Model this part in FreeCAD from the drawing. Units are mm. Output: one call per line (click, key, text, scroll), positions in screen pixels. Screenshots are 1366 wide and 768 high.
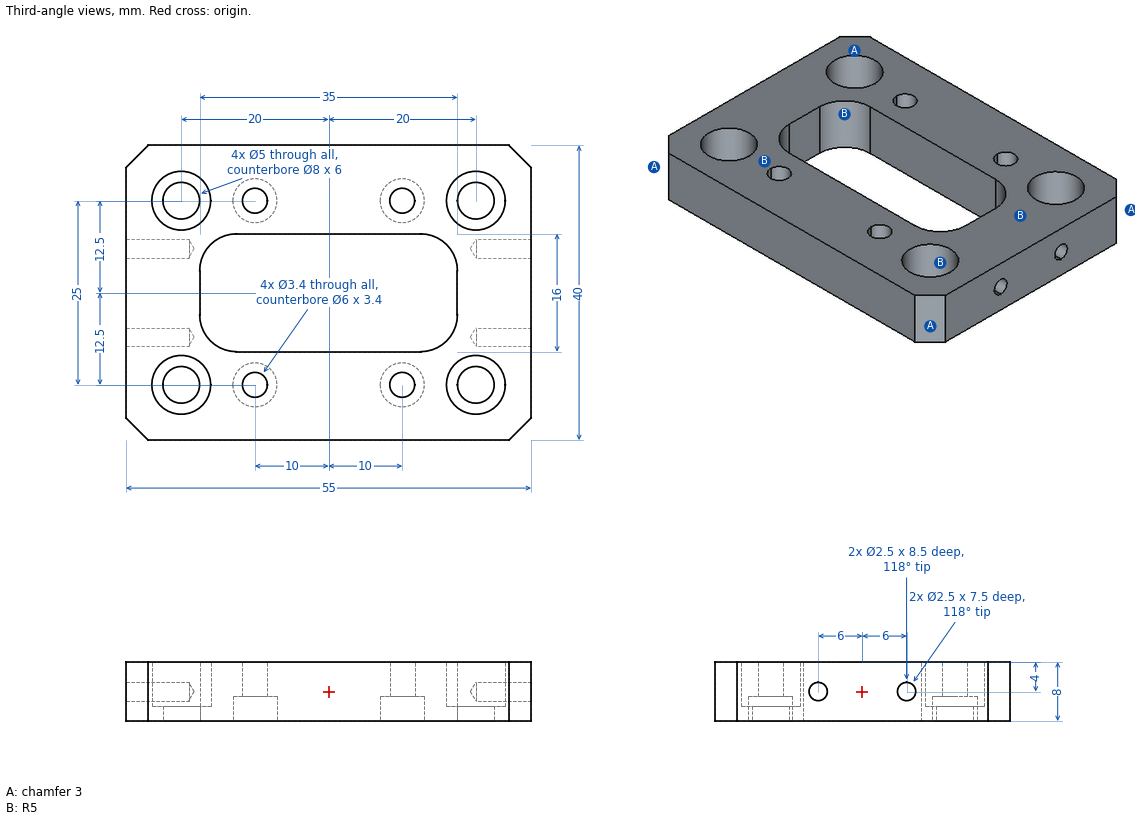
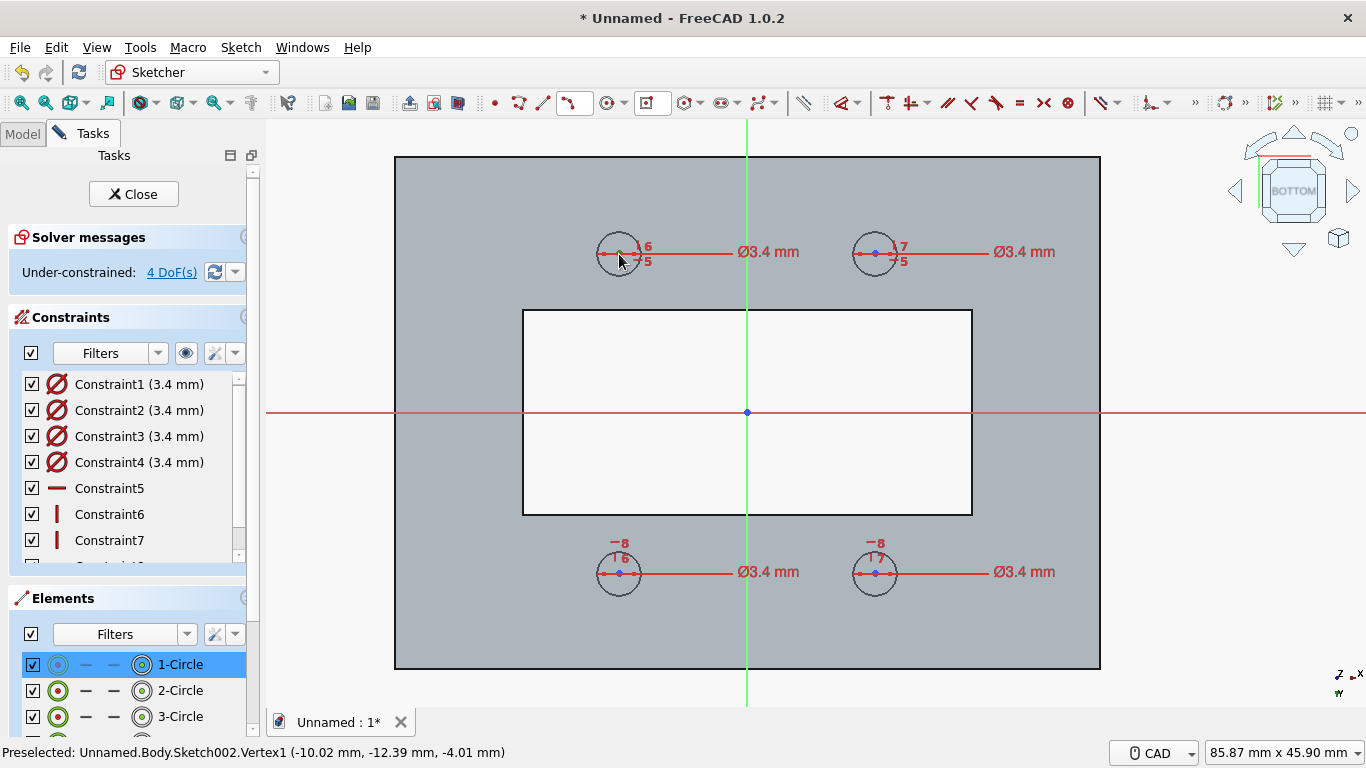
click(860, 104)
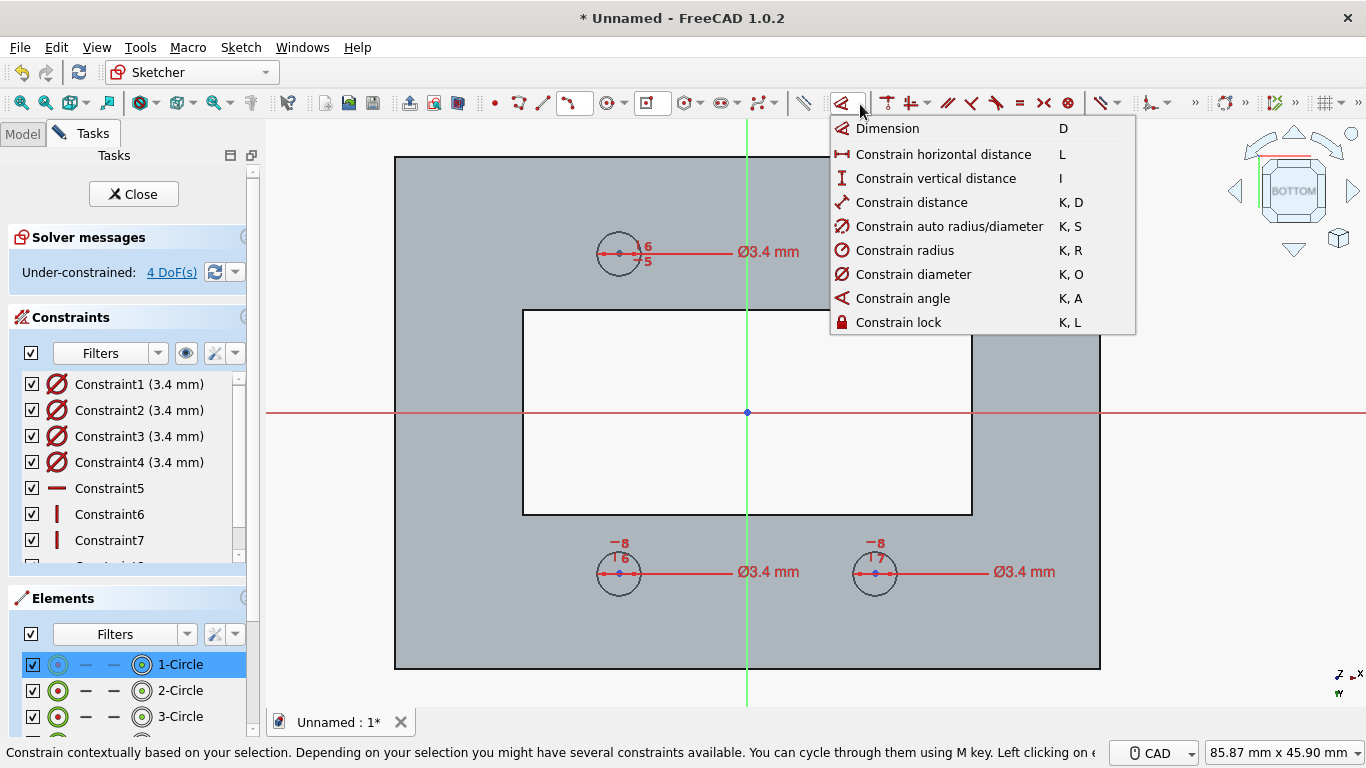
click(983, 154)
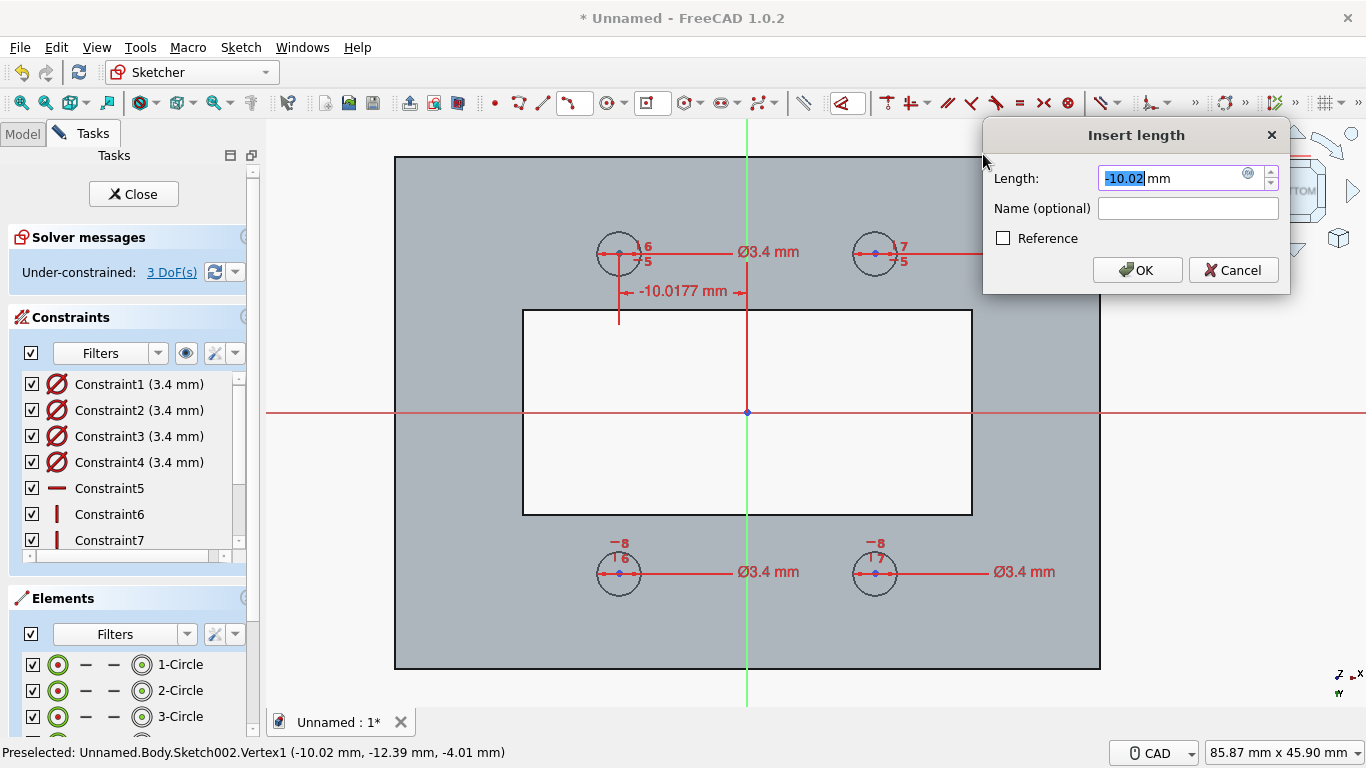
text(-10)
key(Return)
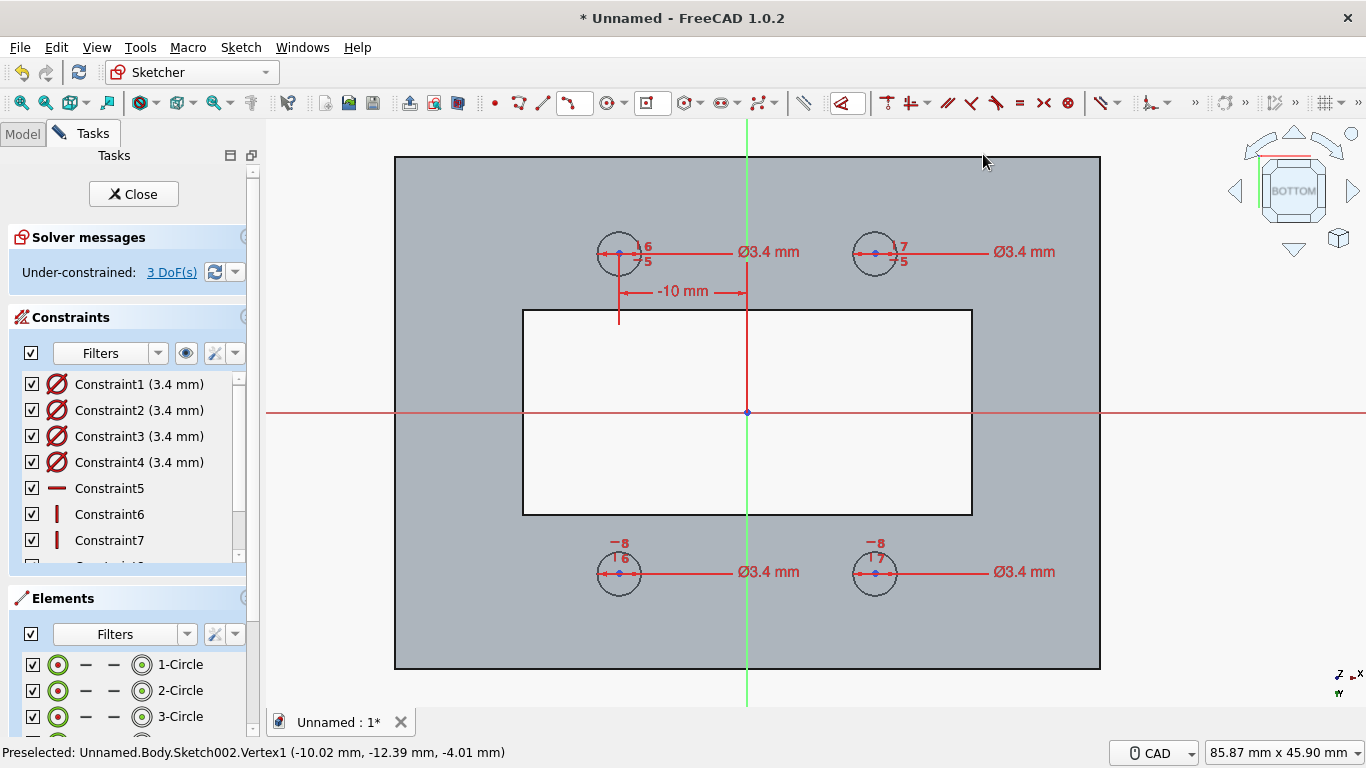
click(875, 254)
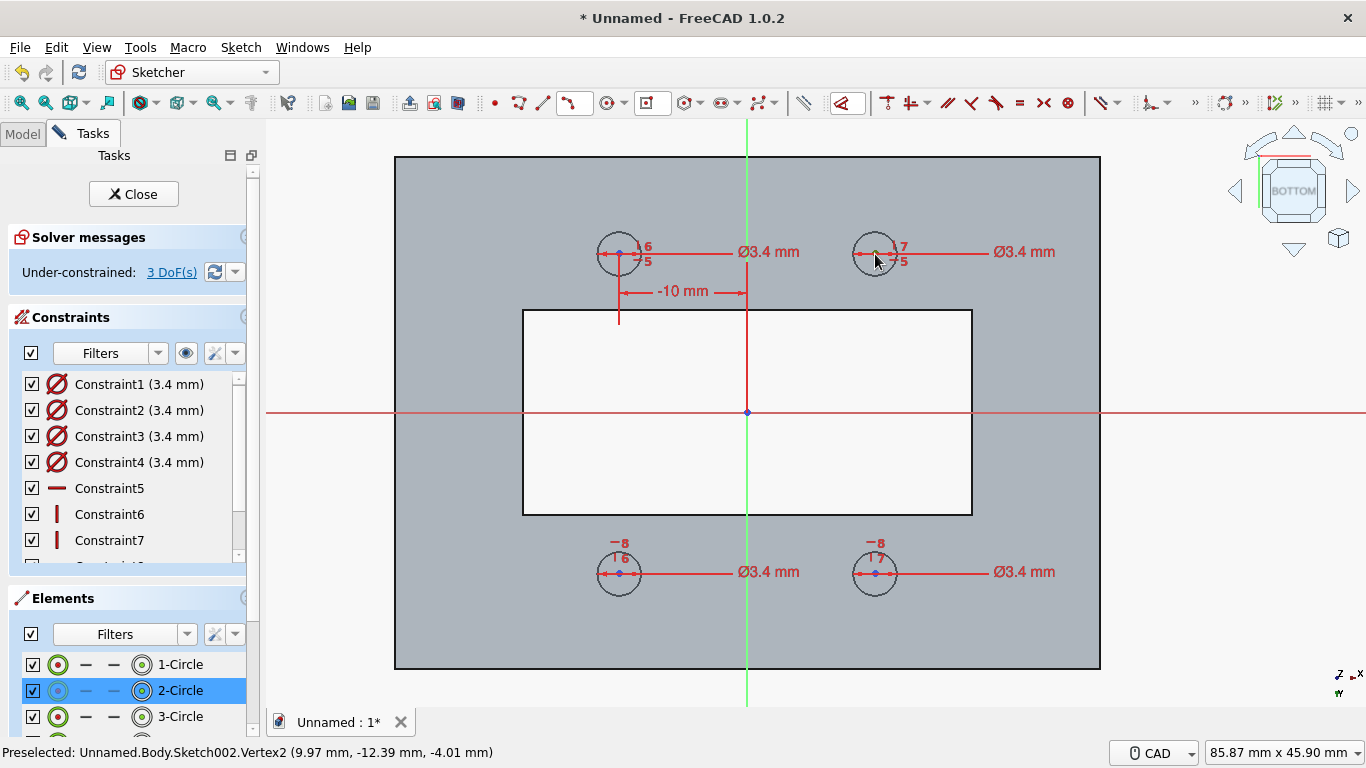
click(860, 104)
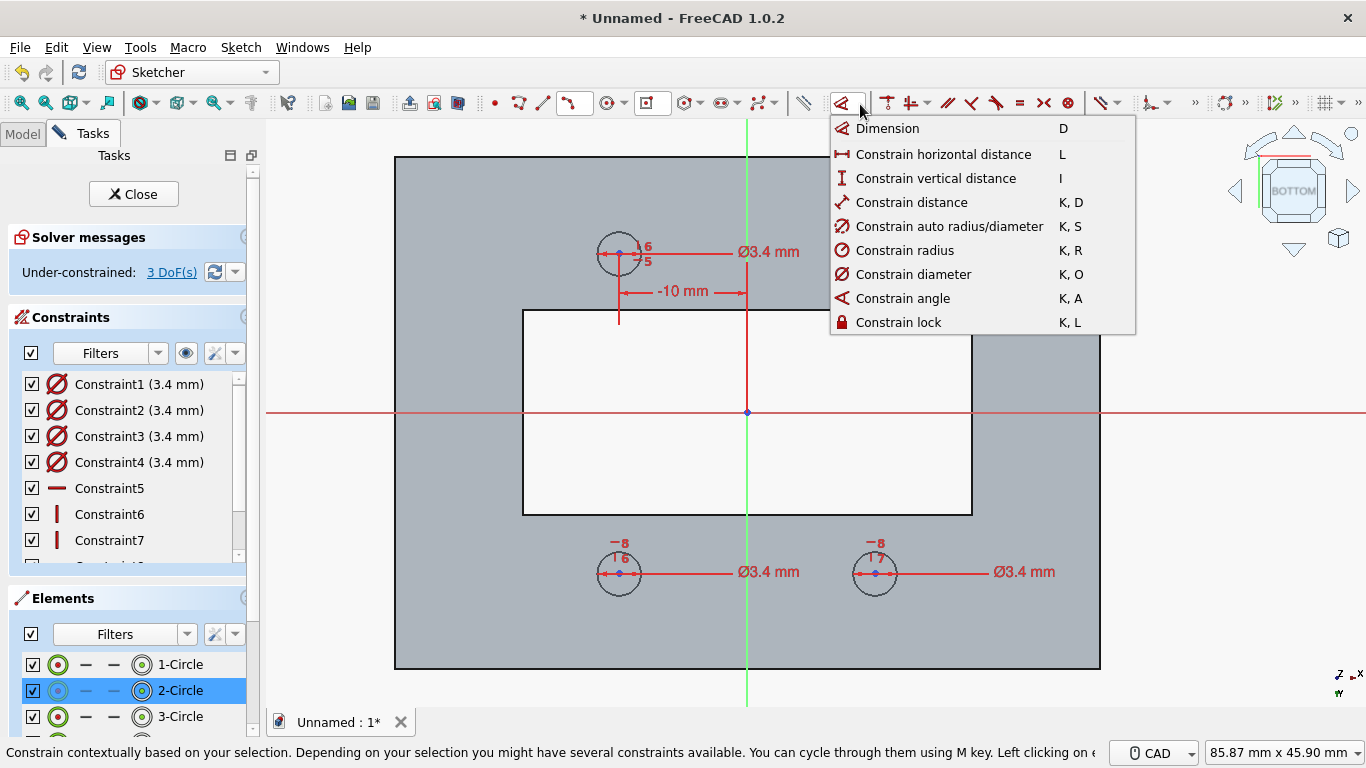
click(983, 154)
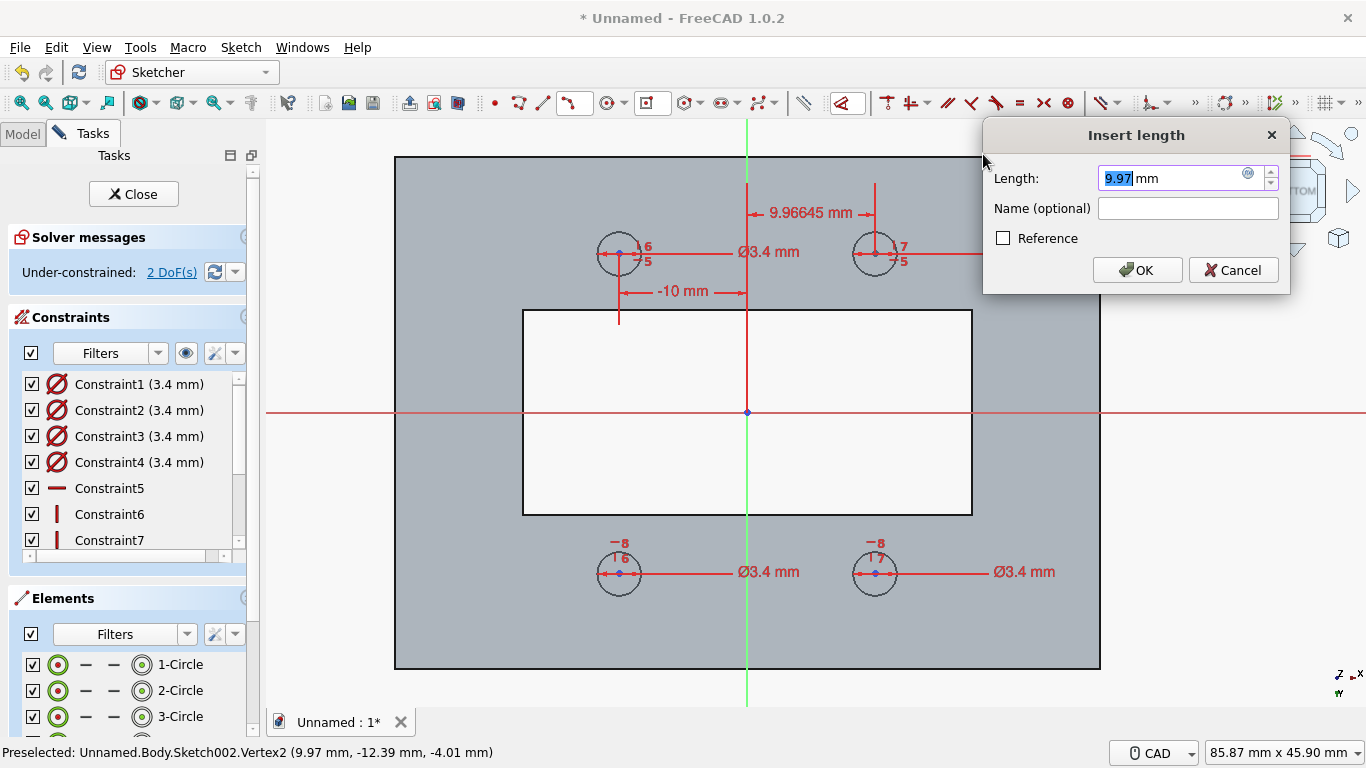
text(10)
key(Return)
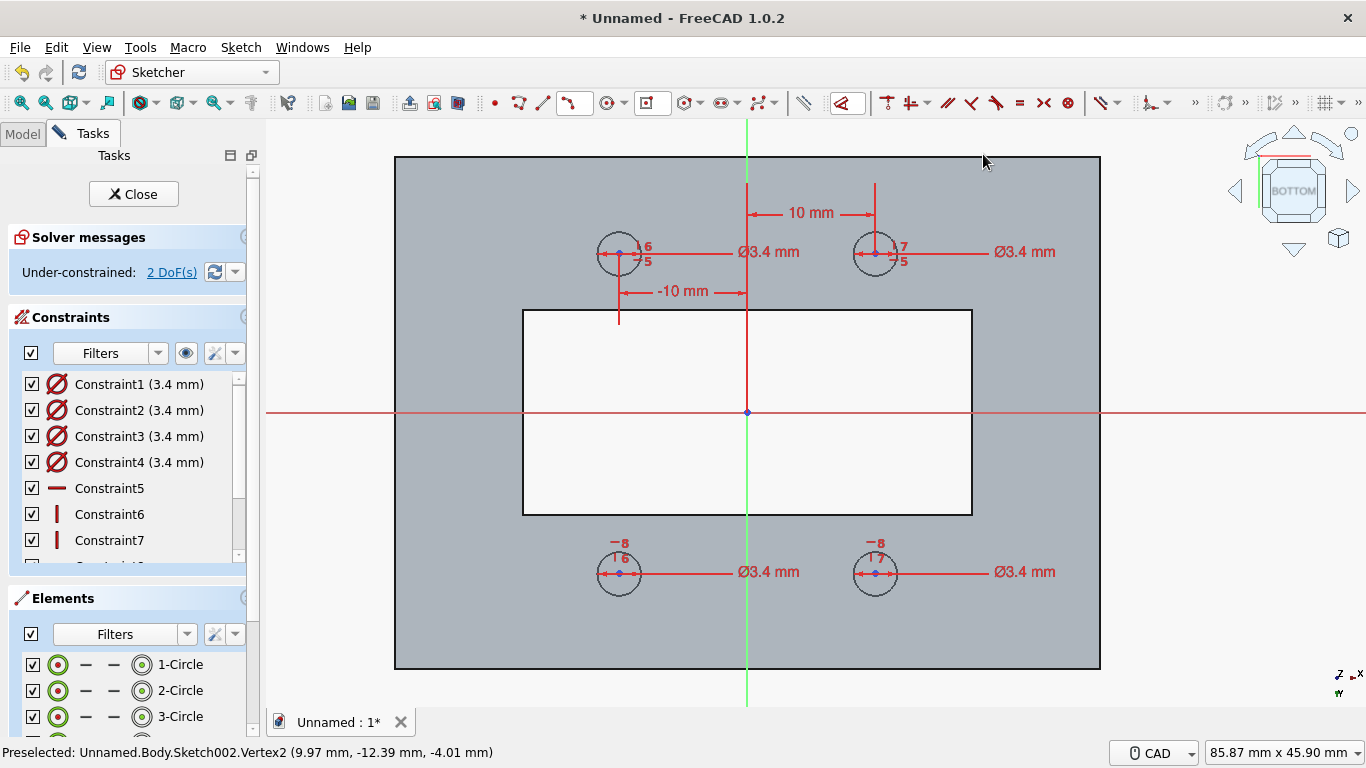
click(619, 254)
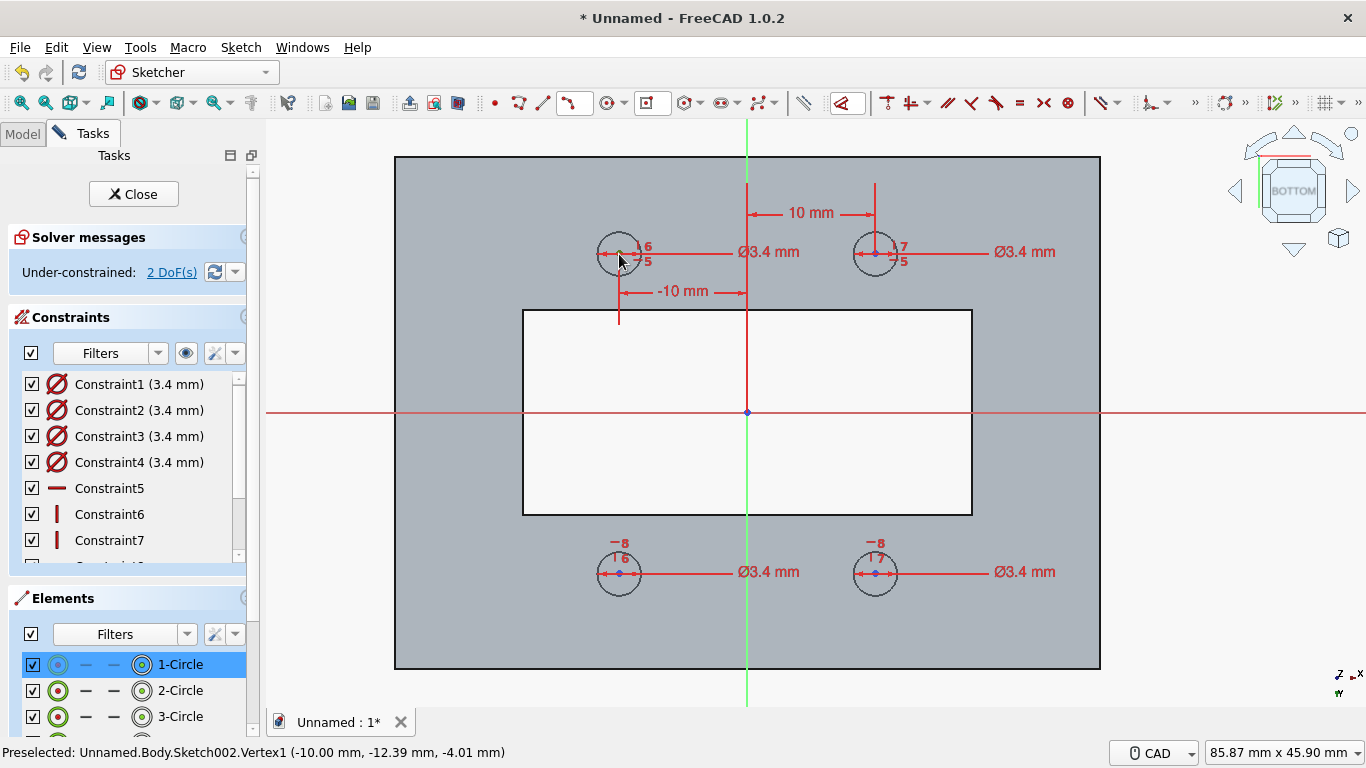
click(619, 574)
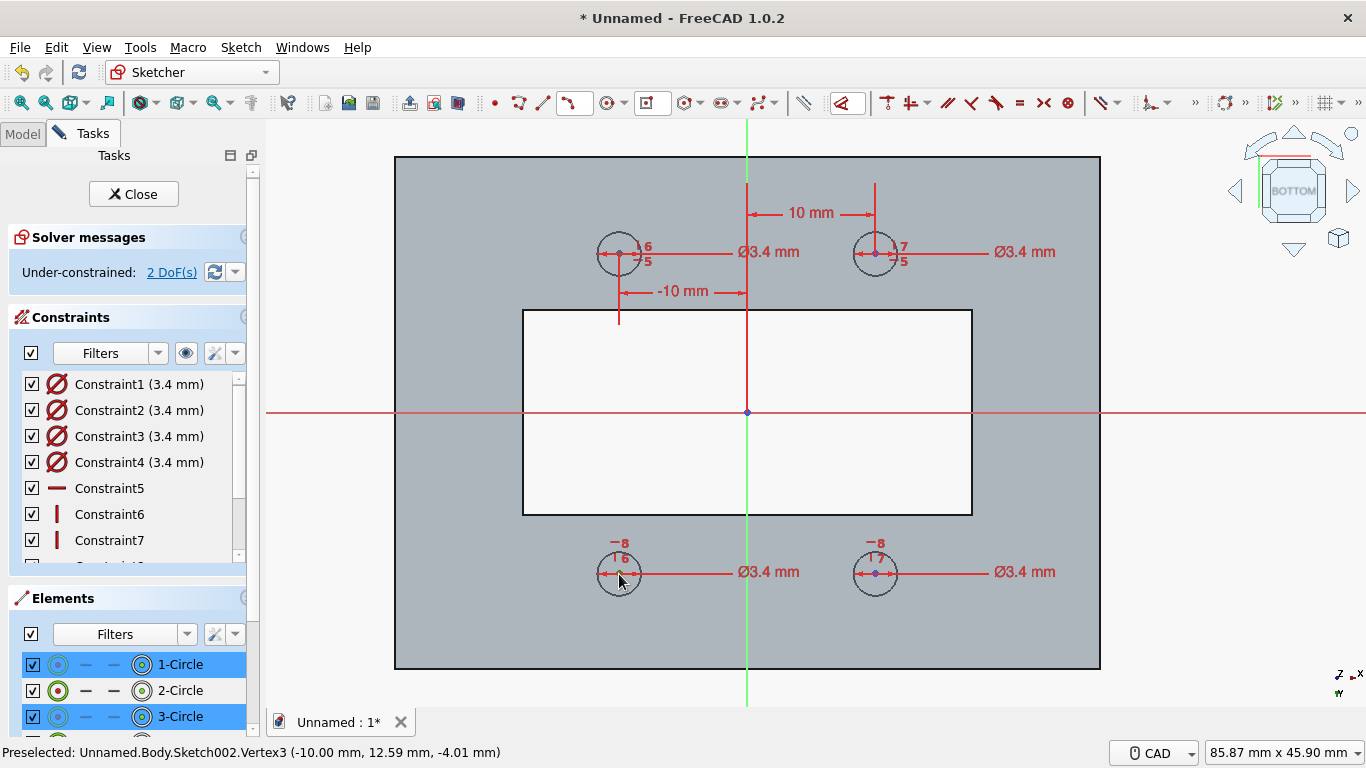
click(860, 104)